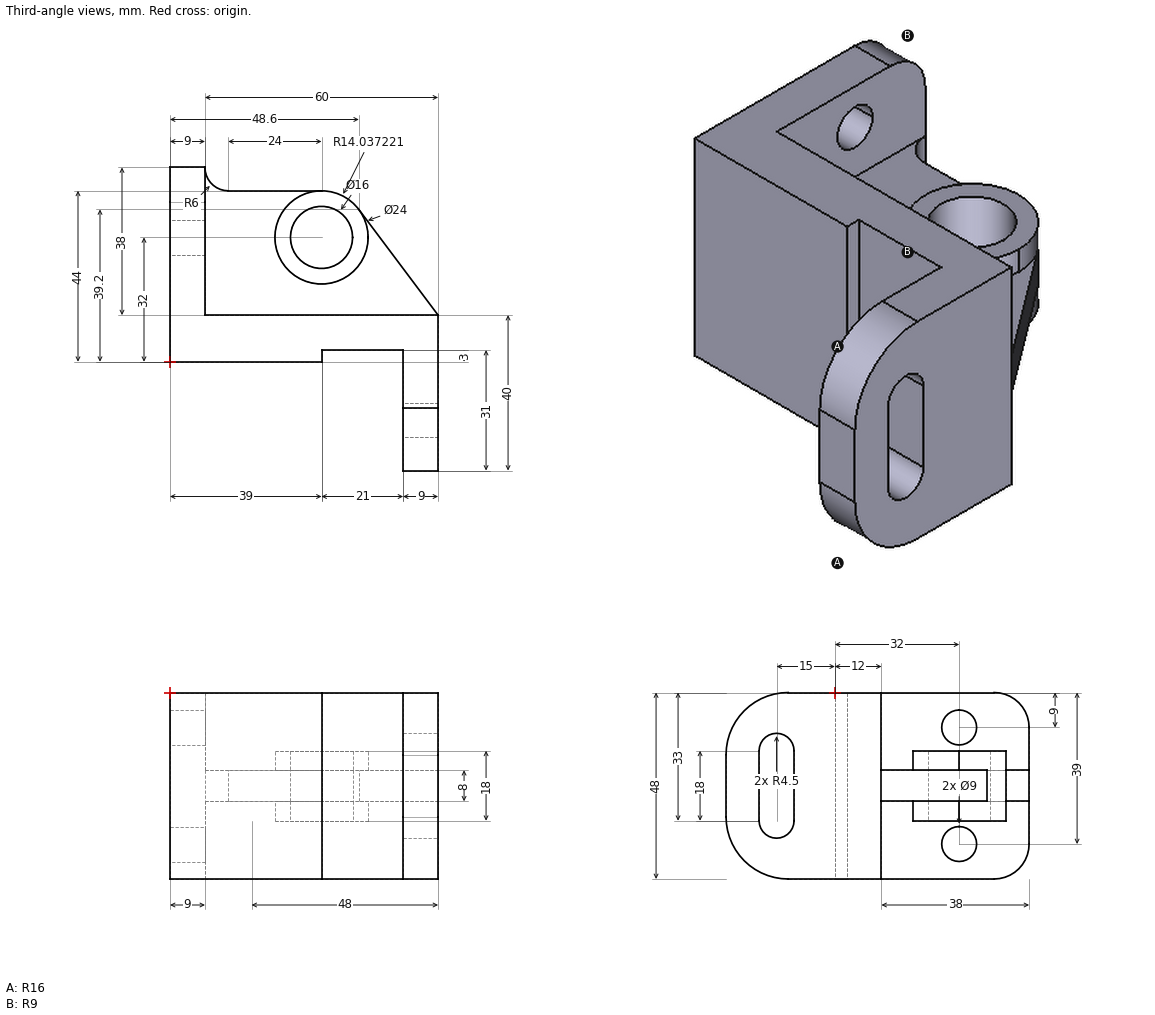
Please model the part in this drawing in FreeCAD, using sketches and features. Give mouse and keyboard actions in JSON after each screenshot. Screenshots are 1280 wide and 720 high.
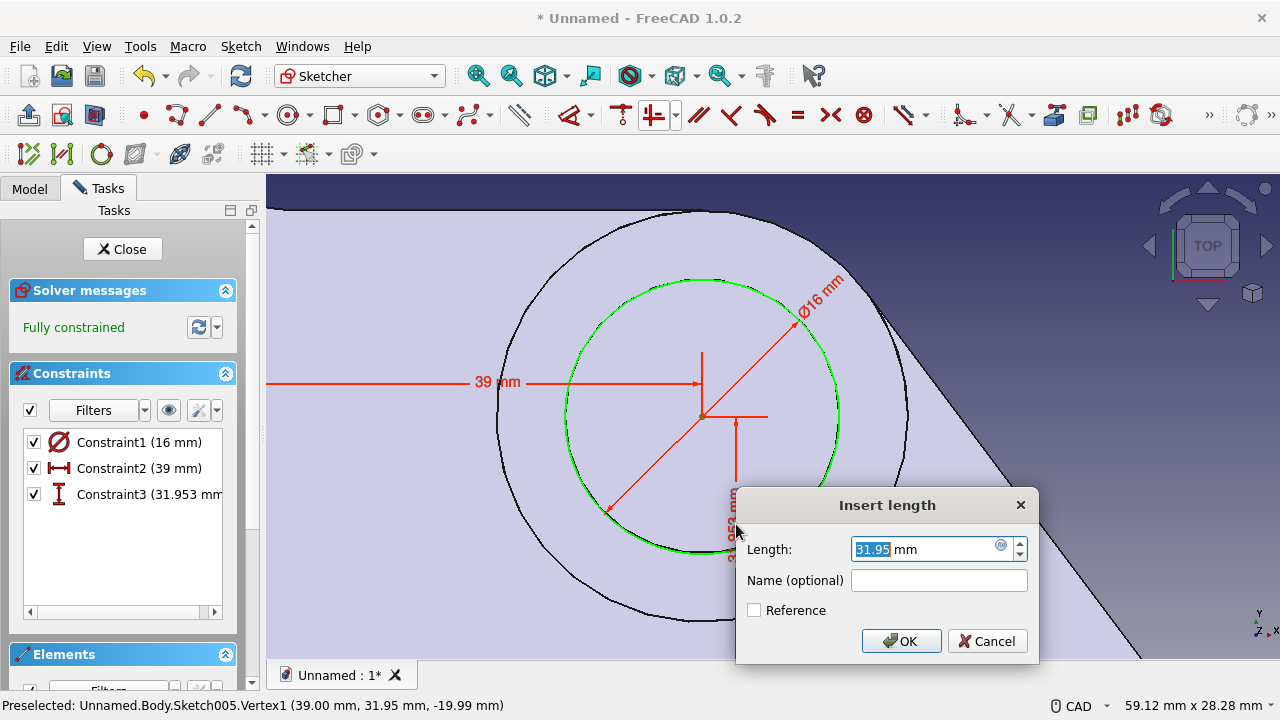
{"action": "type", "text": "32"}
{"action": "key", "text": "Return"}
{"action": "key", "text": "Escape"}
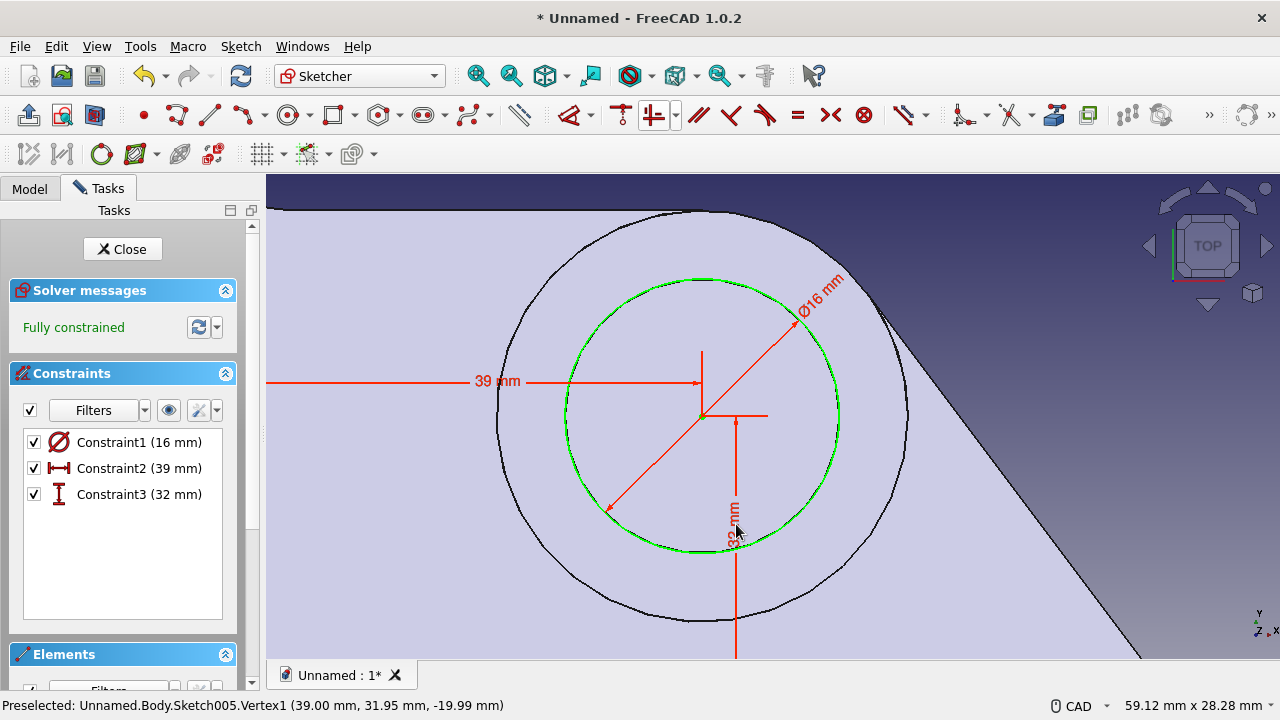
{"action": "left_click", "coordinate": [123, 249]}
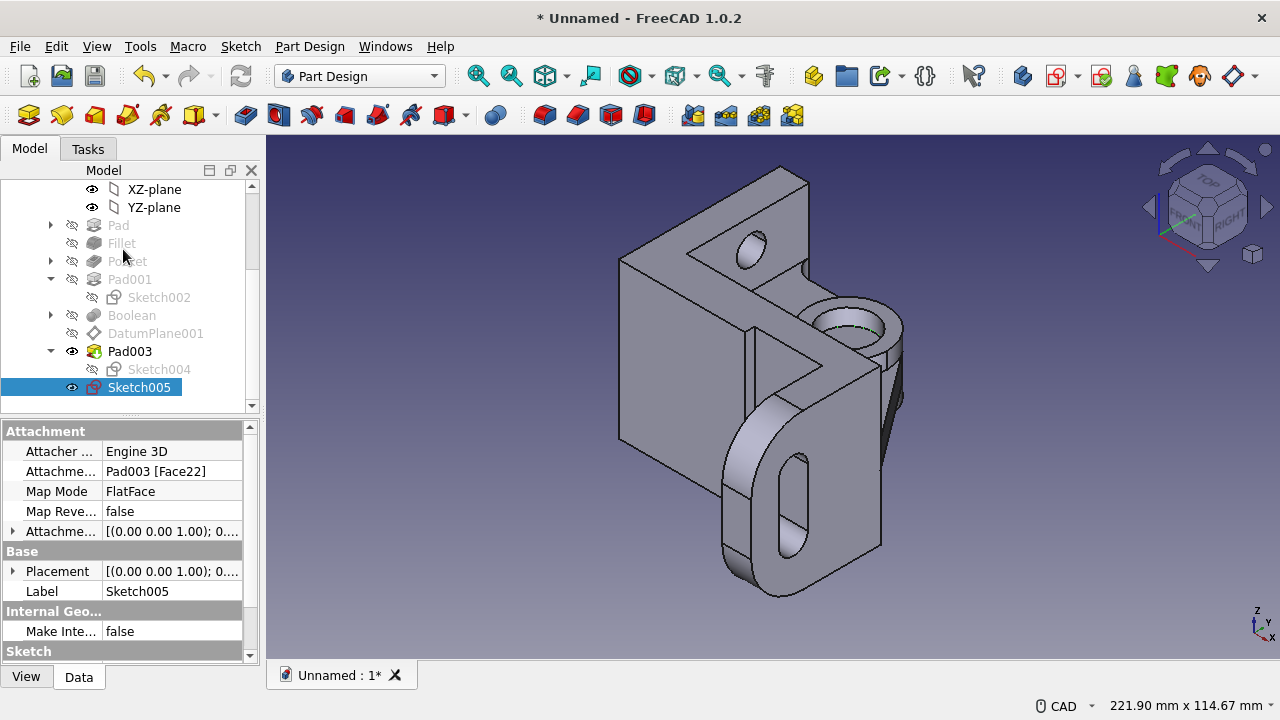
{"action": "left_click", "coordinate": [246, 116]}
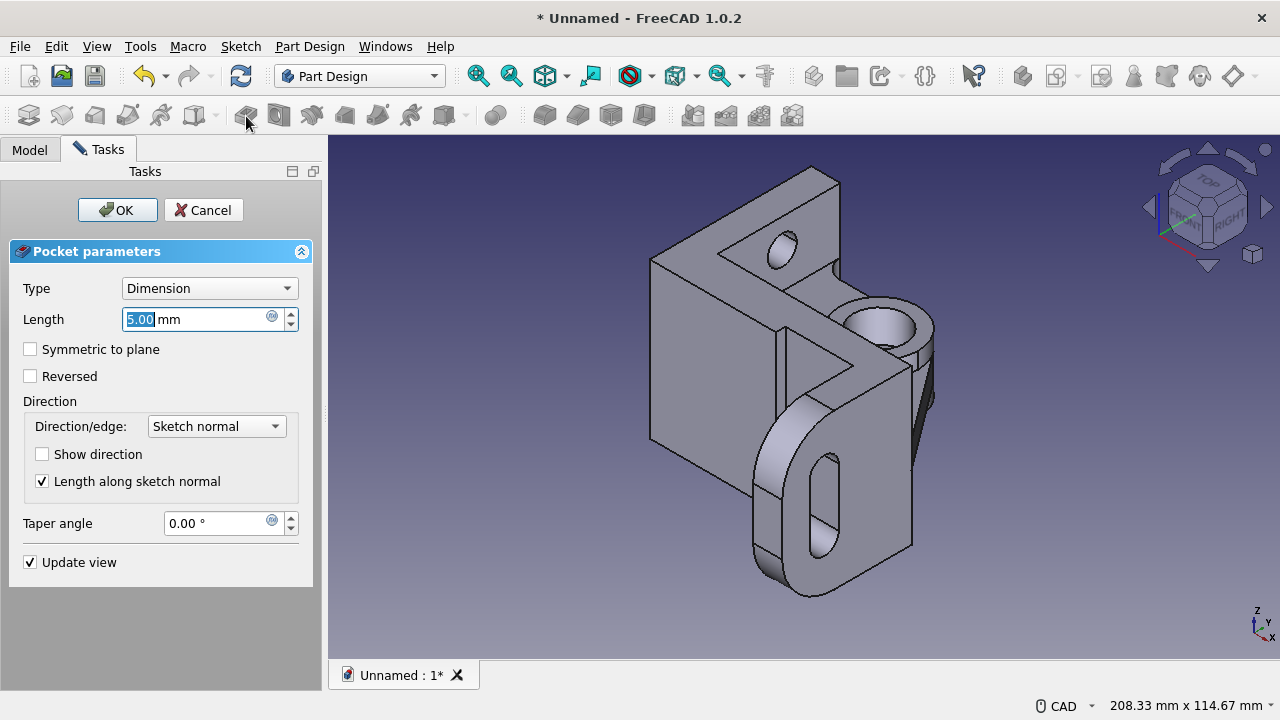
{"action": "left_click", "coordinate": [210, 288]}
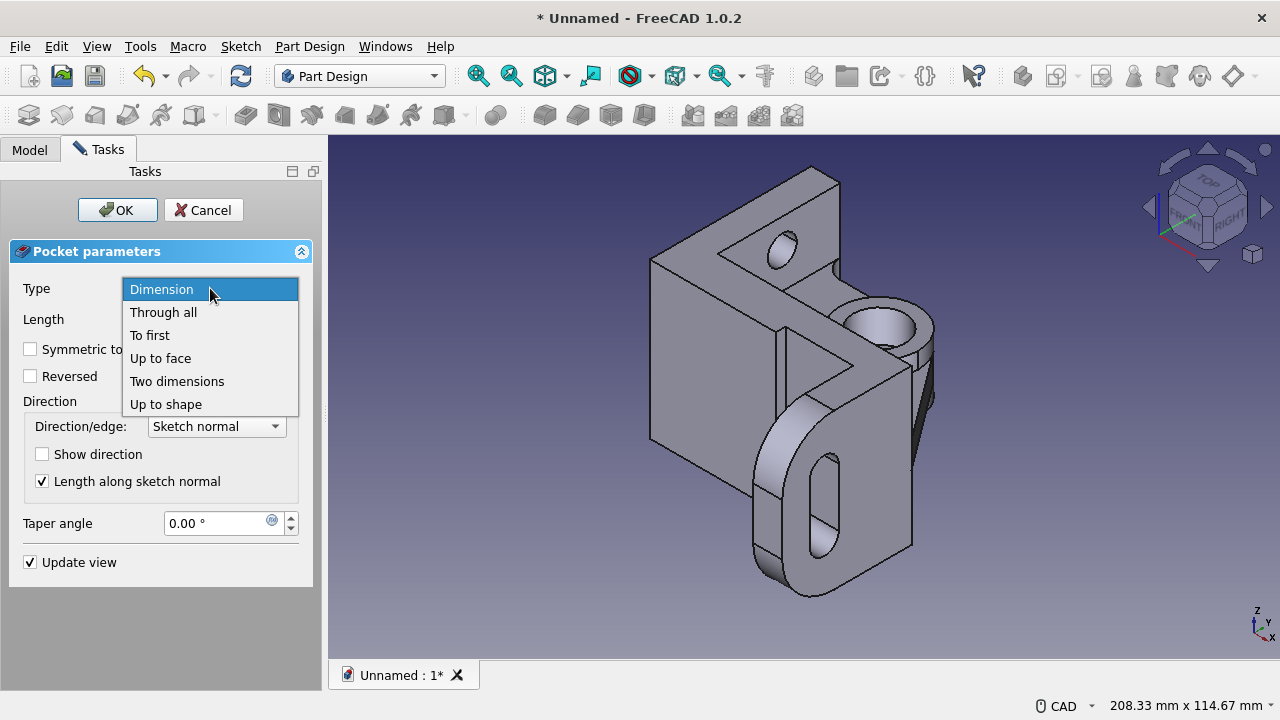
{"action": "left_click", "coordinate": [208, 312]}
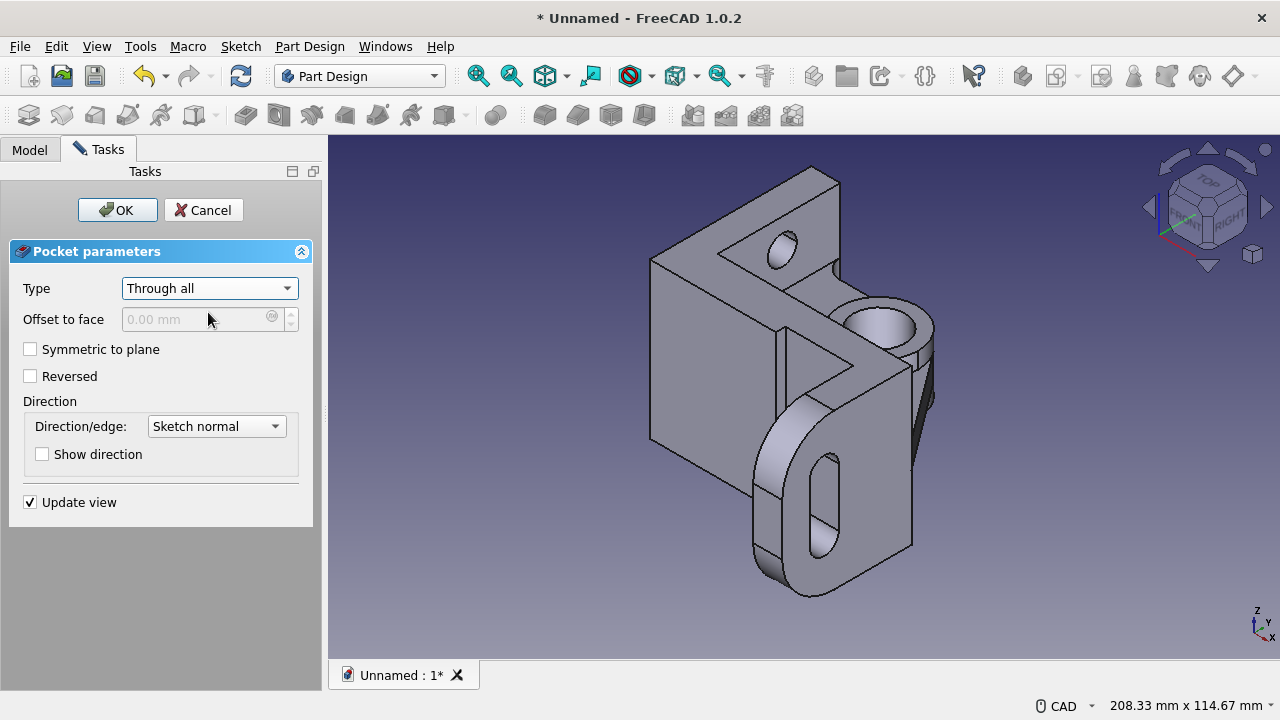
{"action": "left_click", "coordinate": [118, 210]}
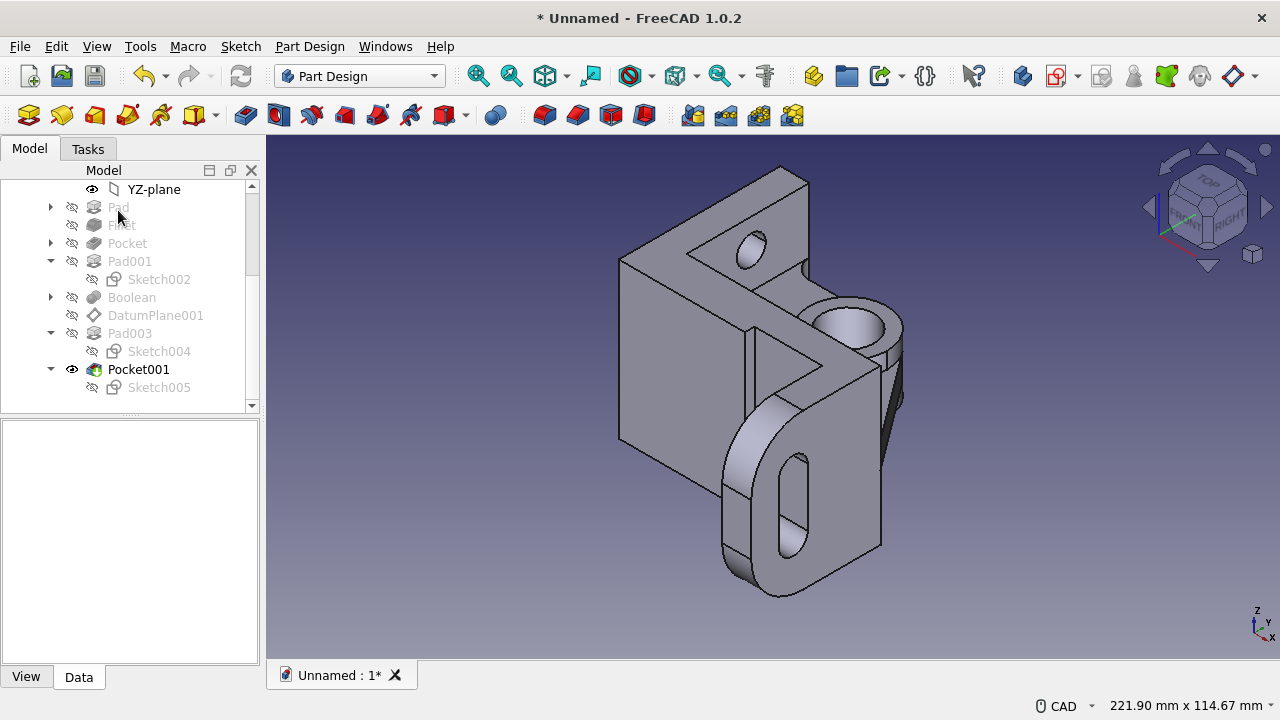
{"action": "key", "text": "2"}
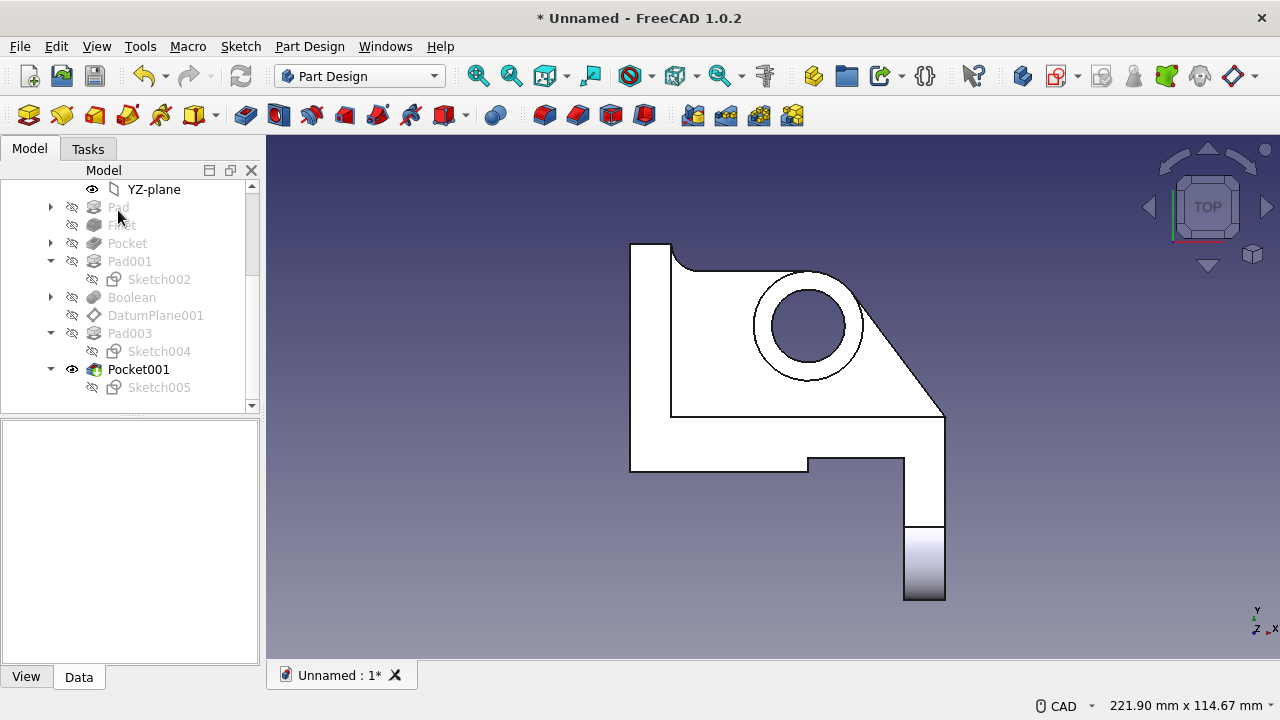
{"action": "left_click", "coordinate": [651, 243]}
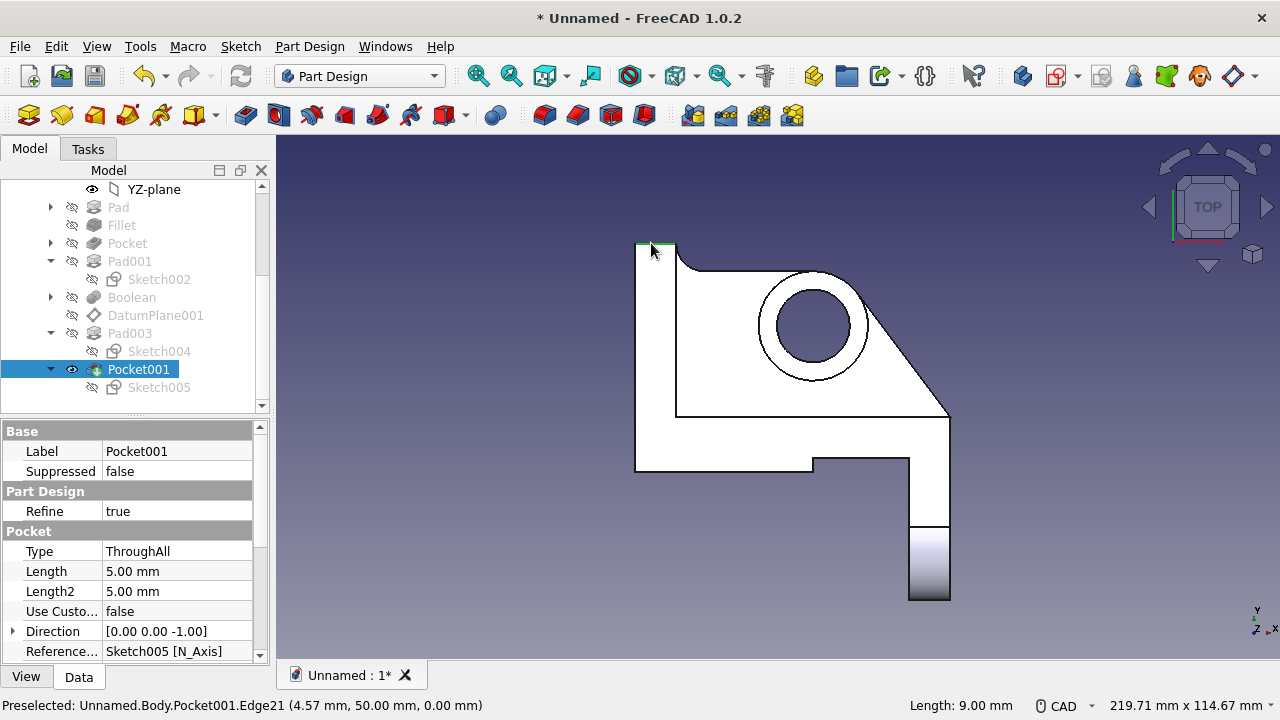
{"action": "key", "text": "0"}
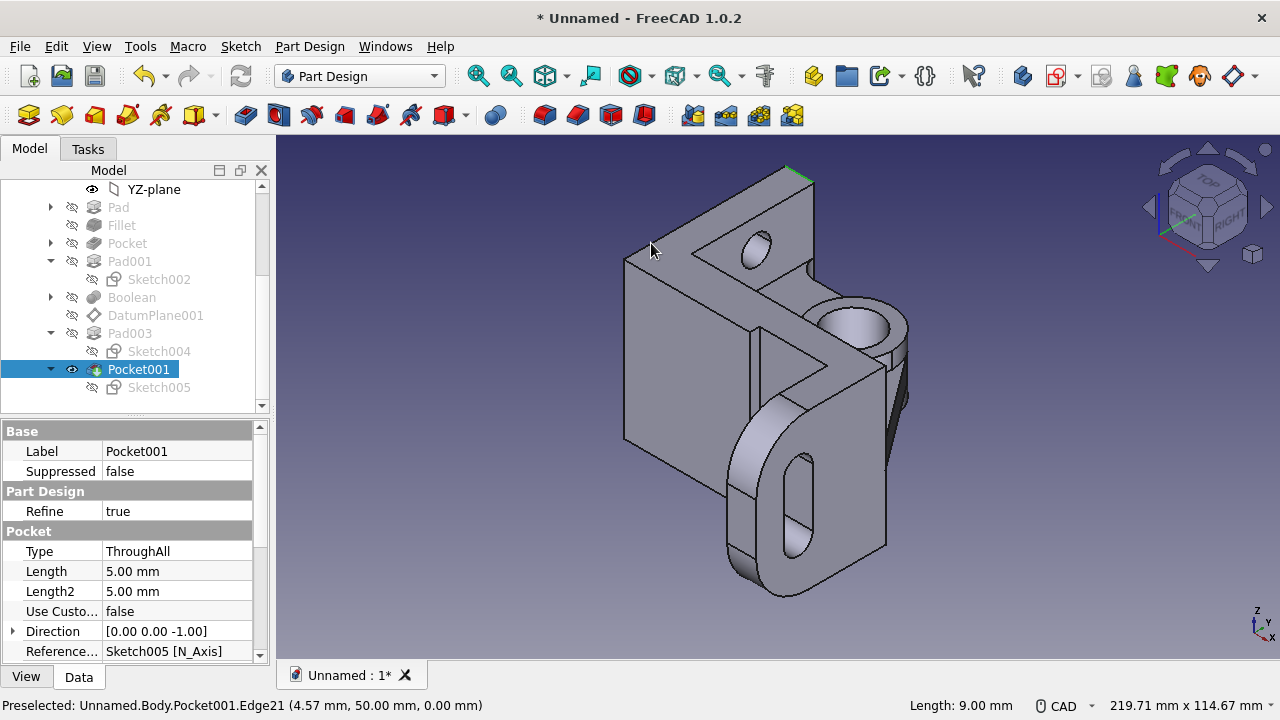
{"action": "key", "text": "1"}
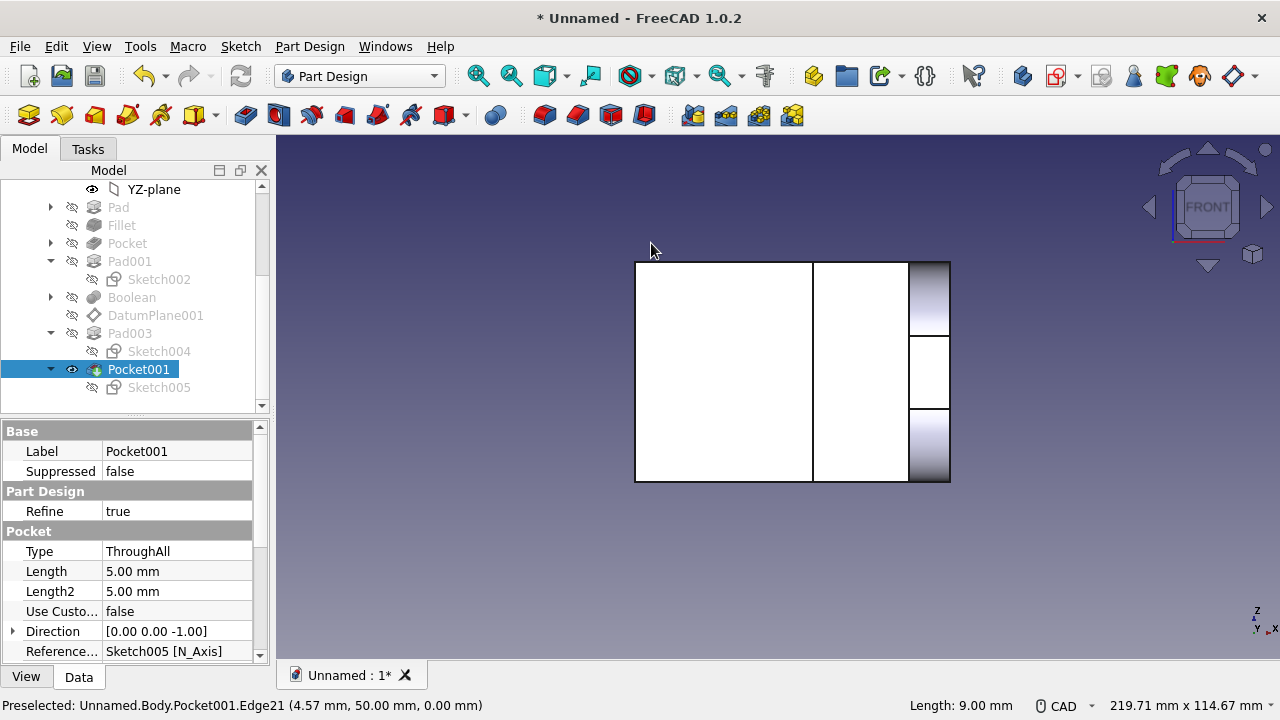
{"action": "key", "text": "v f"}